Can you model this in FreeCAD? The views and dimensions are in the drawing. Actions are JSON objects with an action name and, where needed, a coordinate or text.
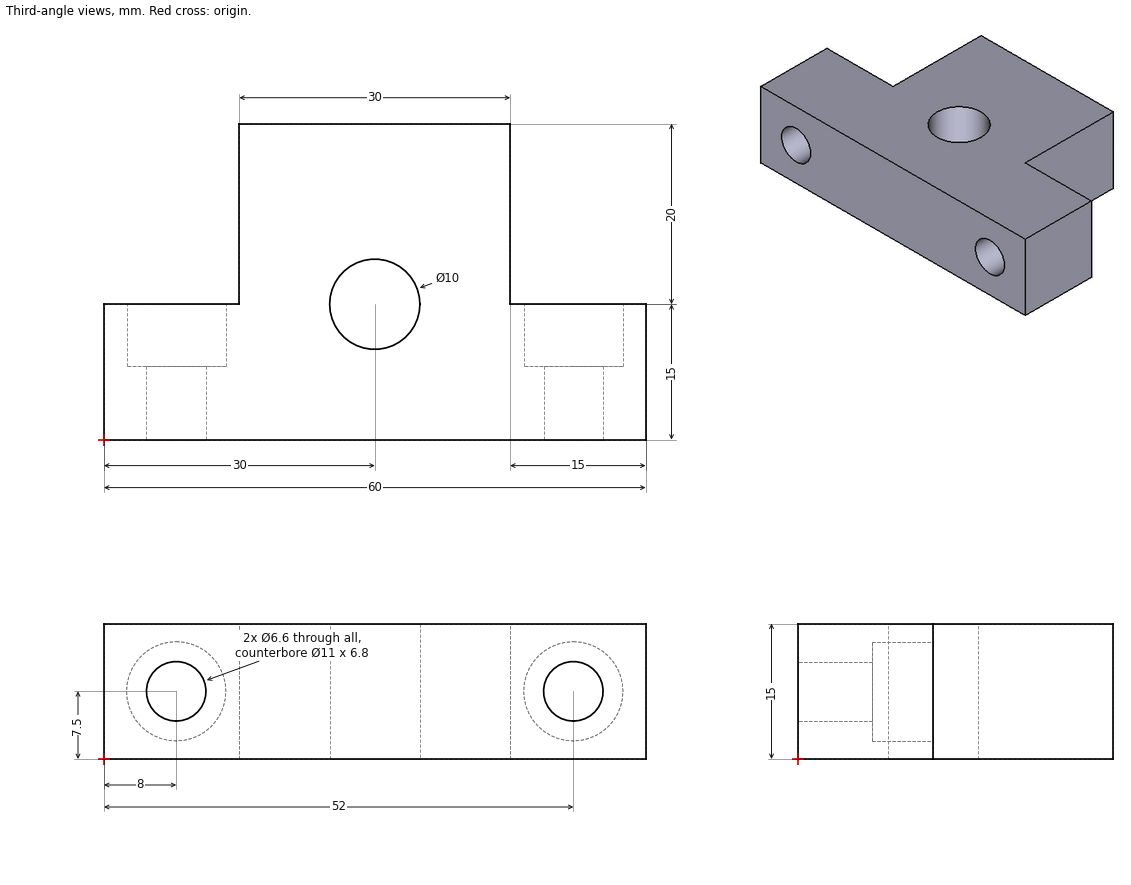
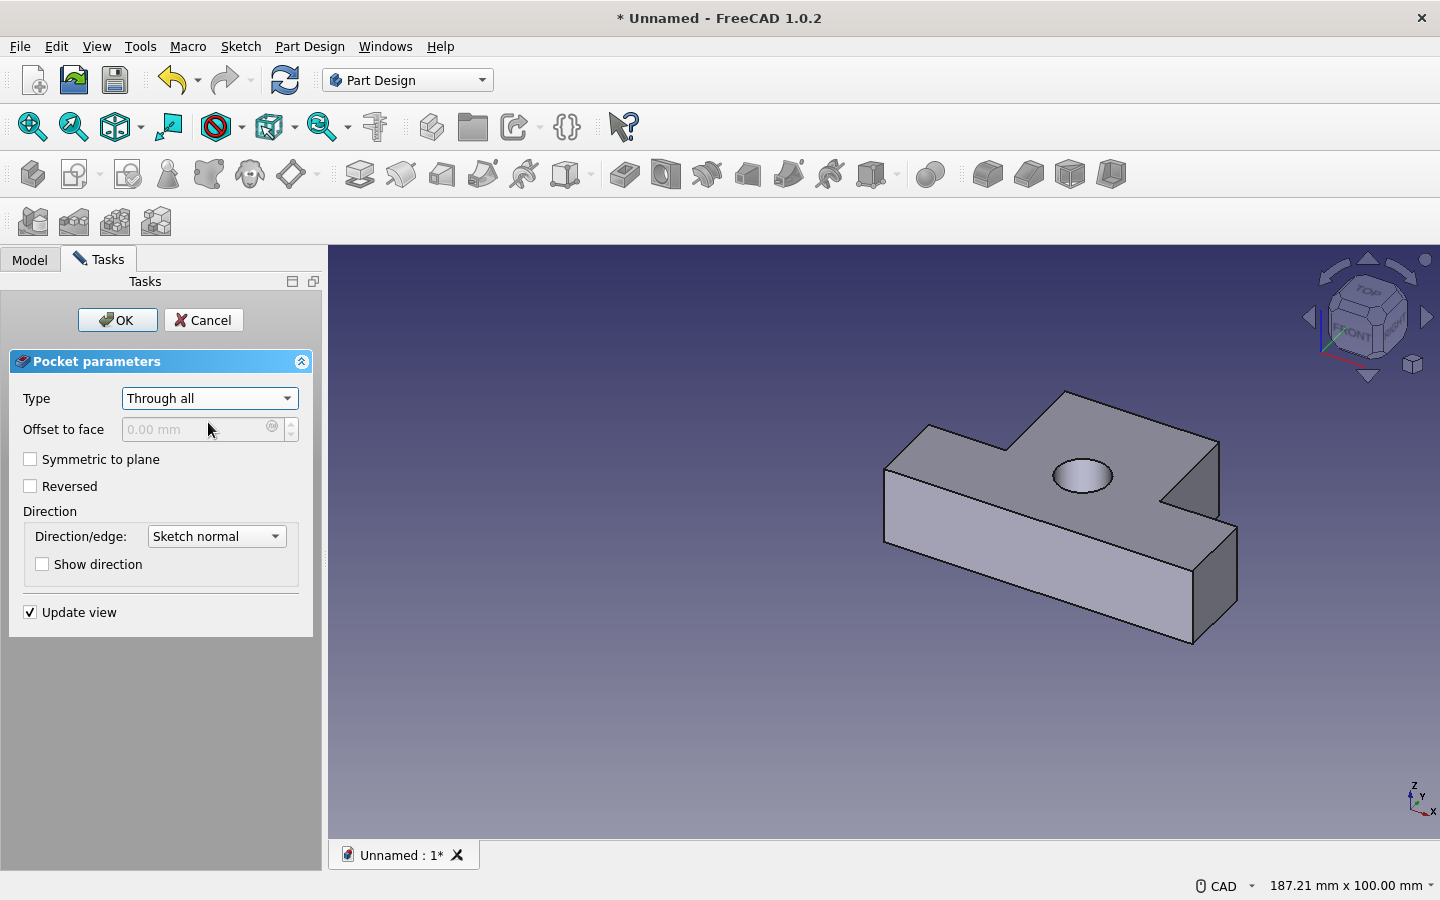
{"action": "left_click", "coordinate": [118, 320]}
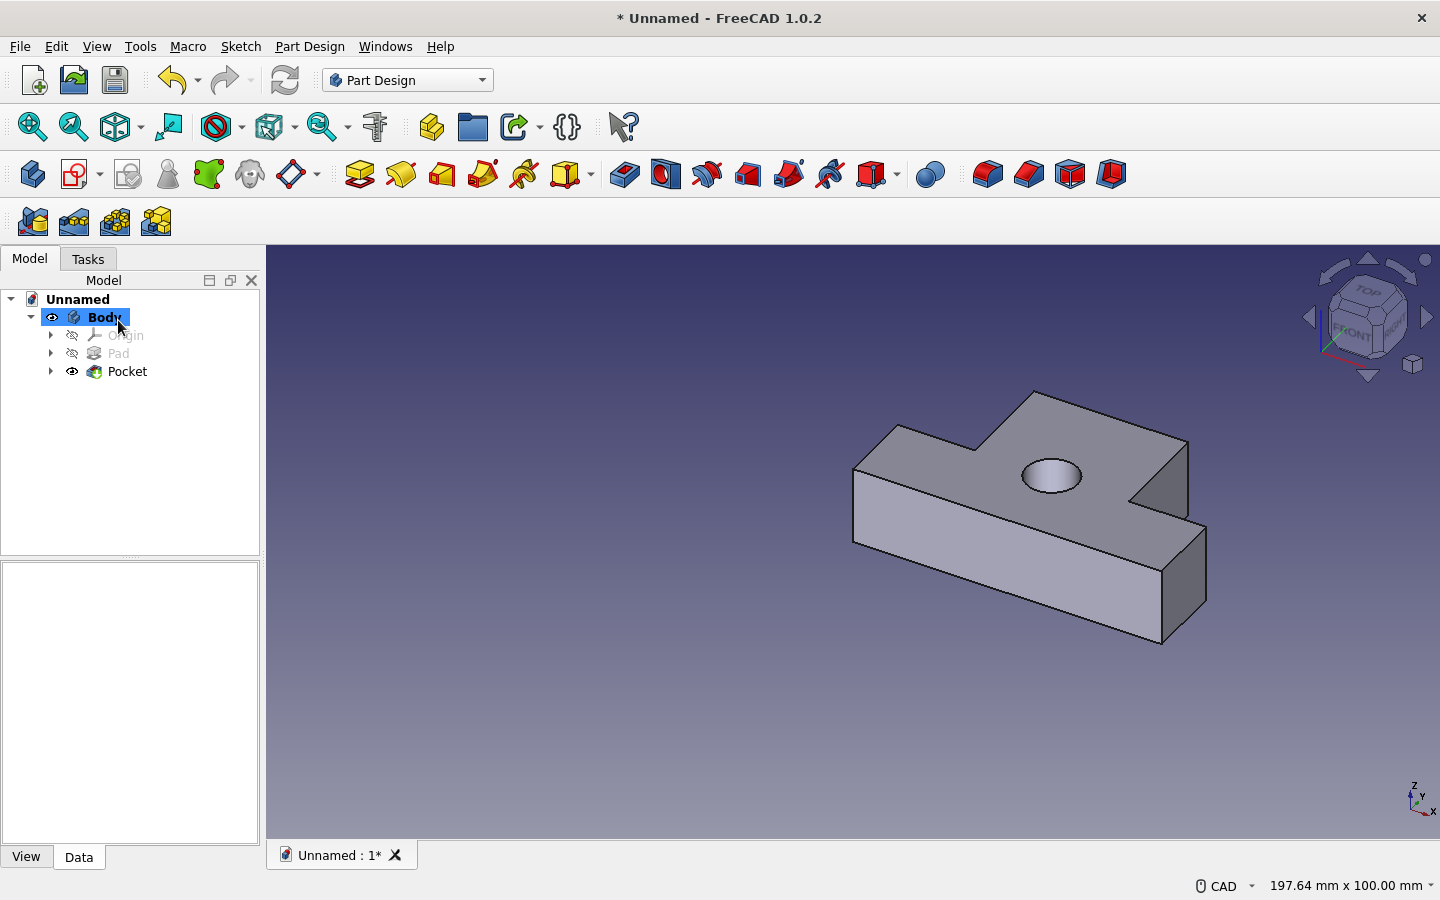
{"action": "key", "text": "4"}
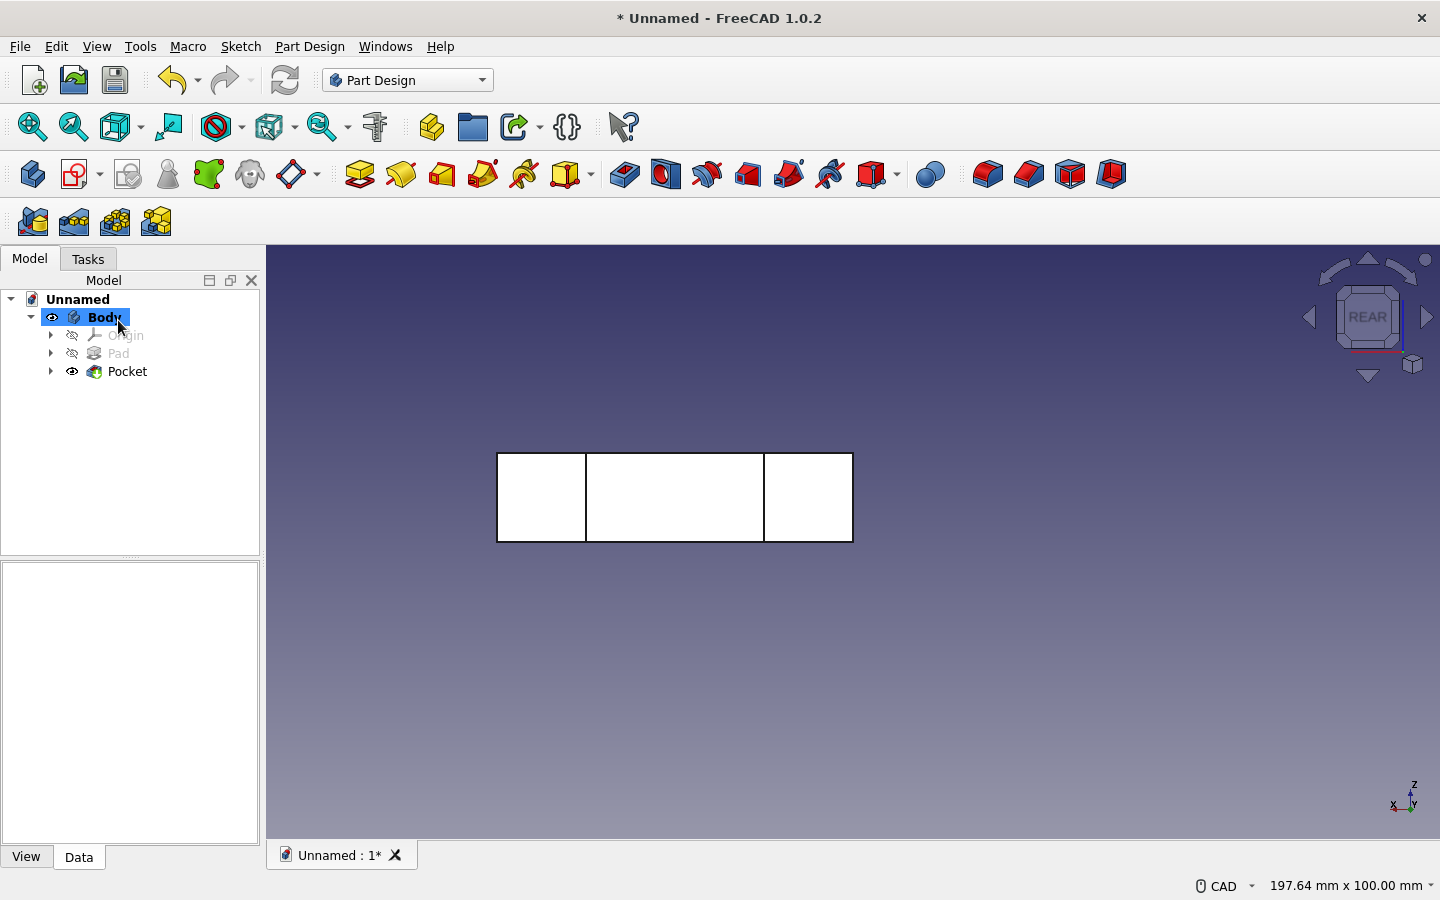
{"action": "left_click", "coordinate": [33, 128]}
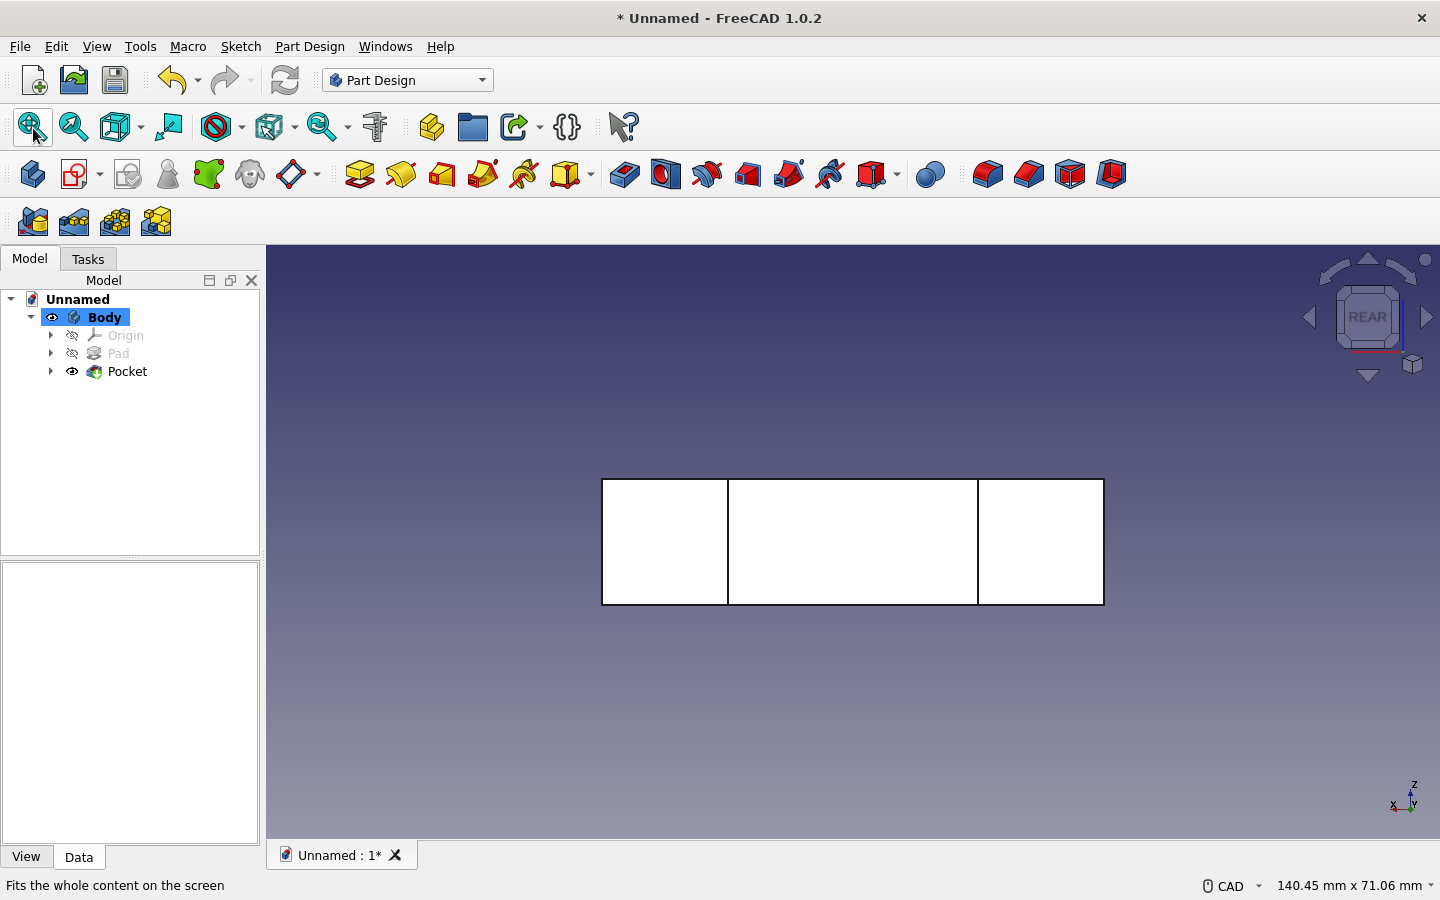
{"action": "left_click", "coordinate": [665, 541]}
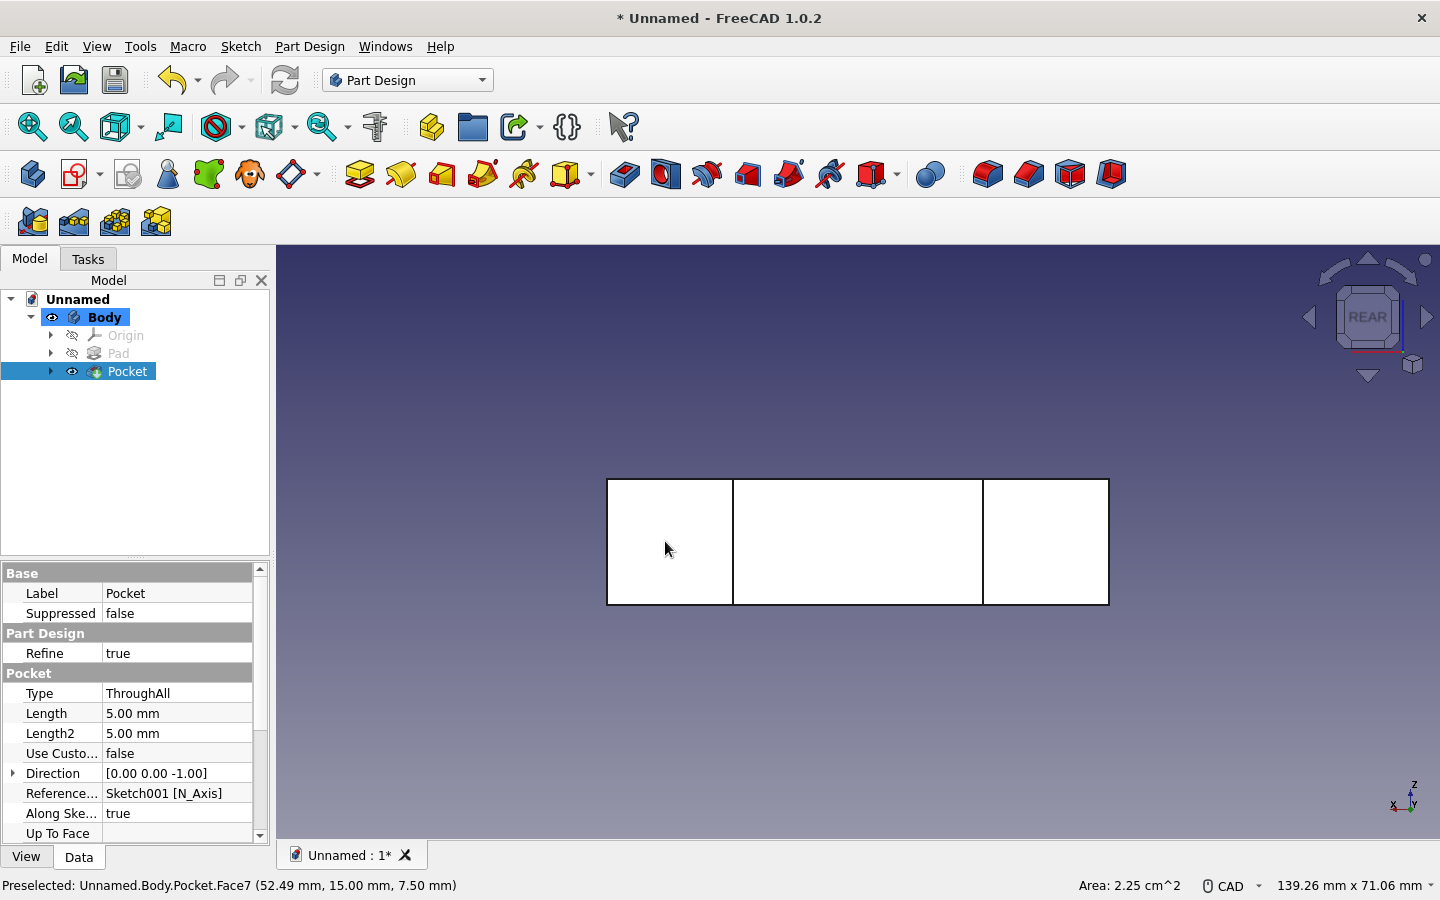
{"action": "left_click", "coordinate": [74, 174]}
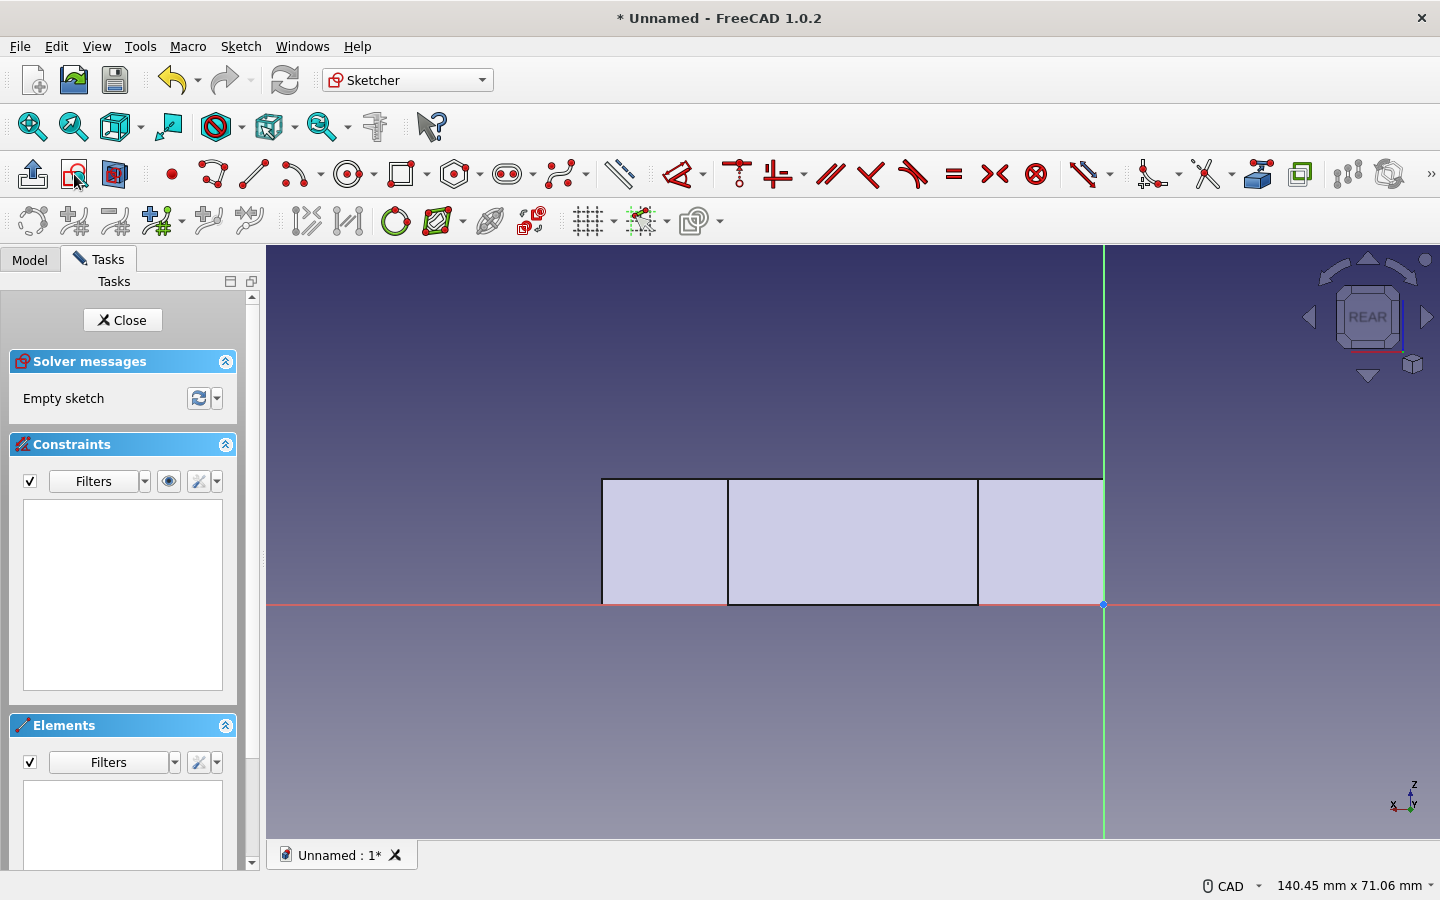
{"action": "left_click", "coordinate": [115, 174]}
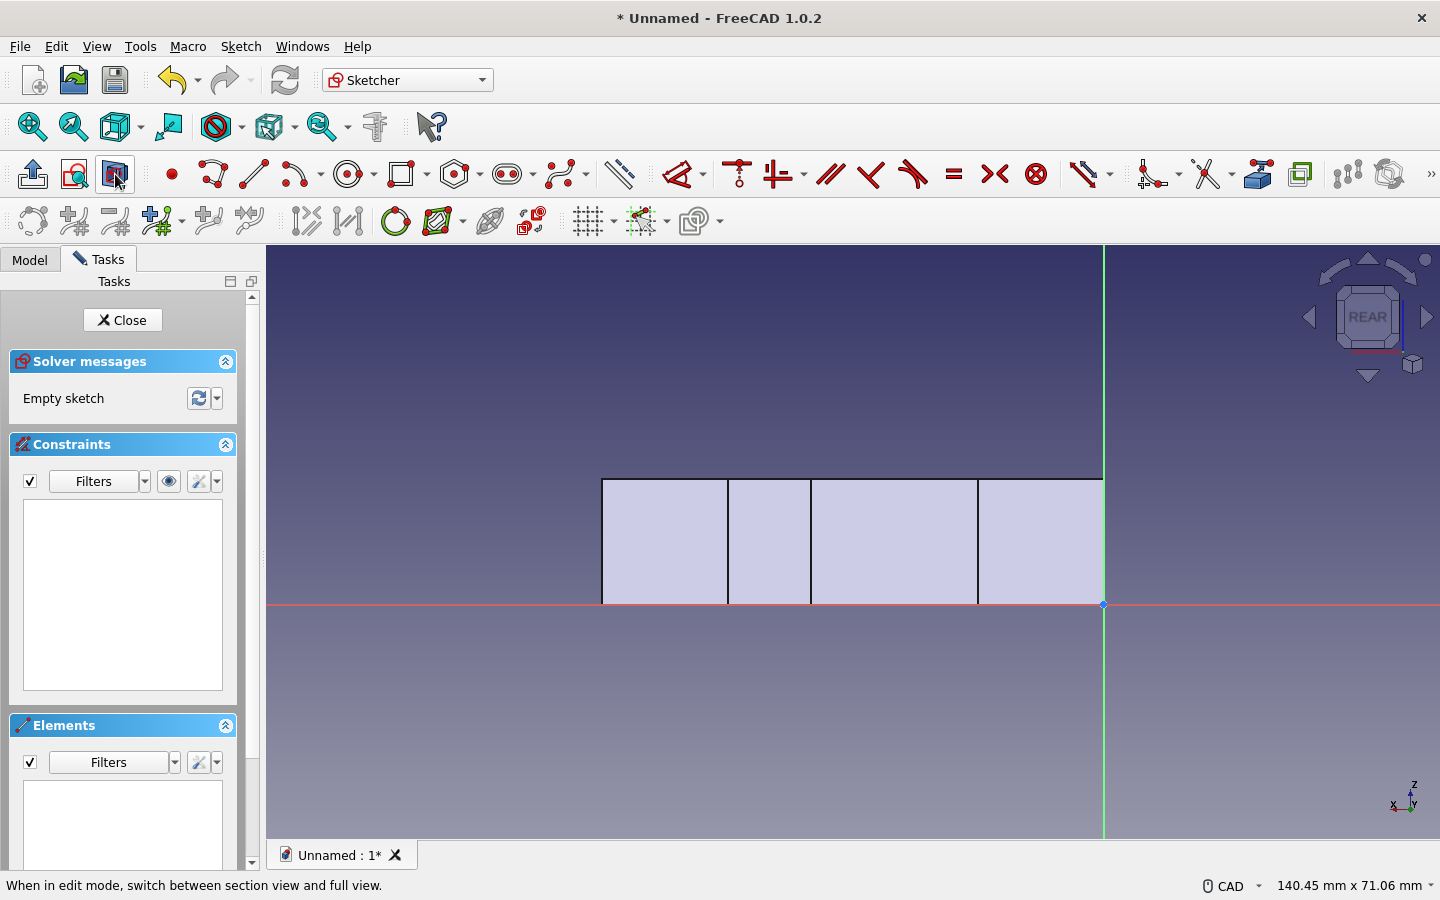
{"action": "scroll", "coordinate": [1052, 595], "scroll_direction": "up", "scroll_amount": 2}